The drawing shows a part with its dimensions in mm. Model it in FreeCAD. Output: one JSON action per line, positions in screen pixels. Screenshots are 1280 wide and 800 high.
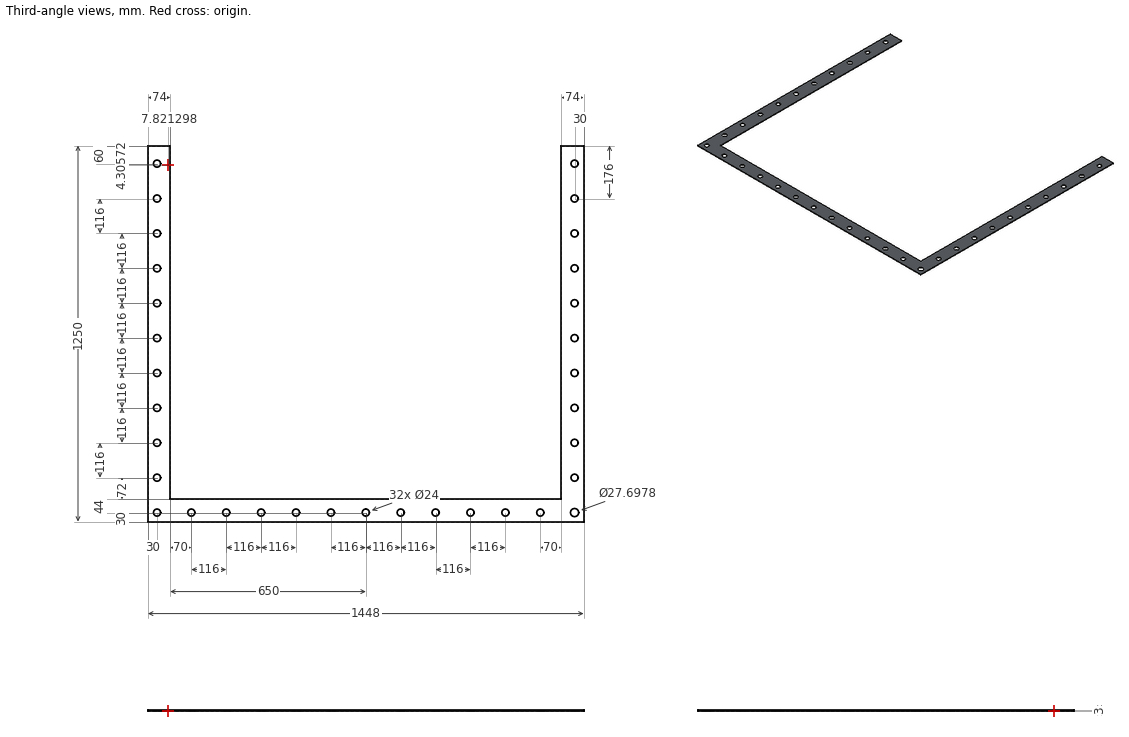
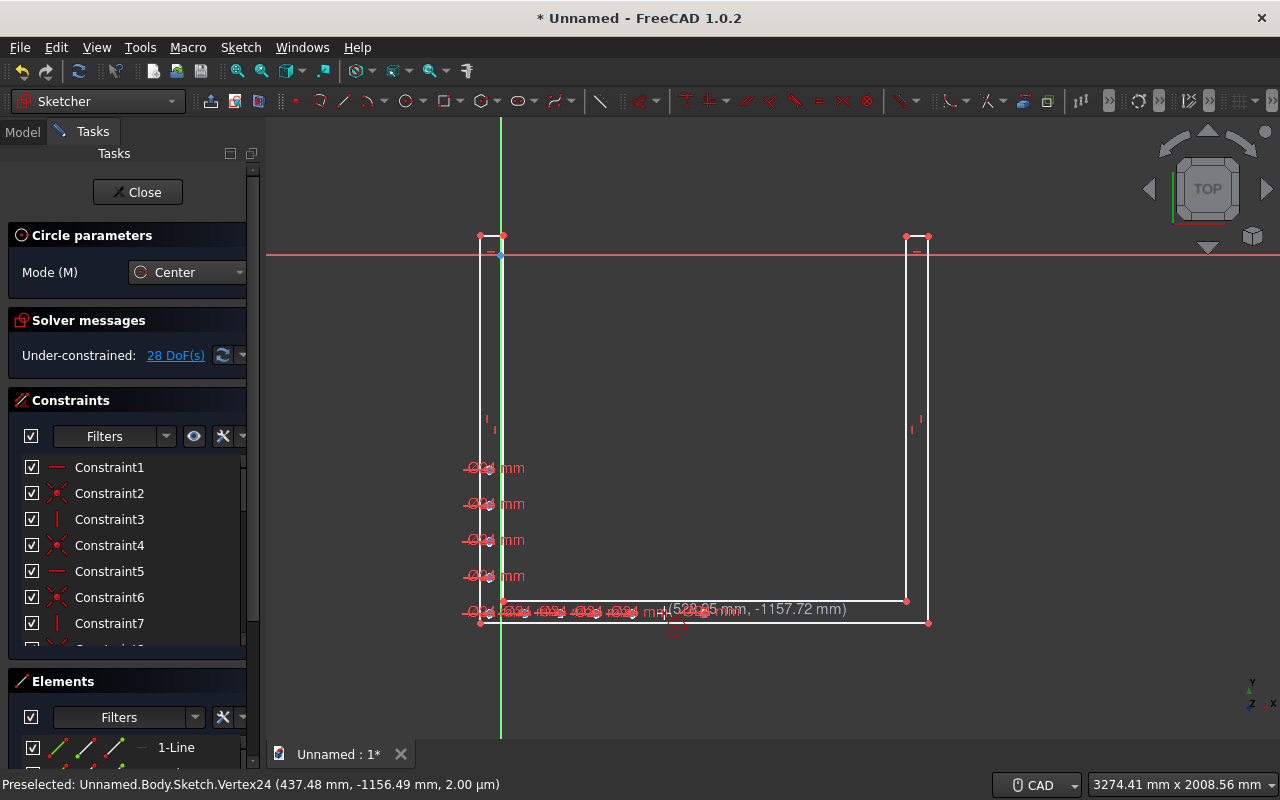
{"action": "scroll", "coordinate": [669, 613], "scroll_direction": "up", "scroll_amount": 3}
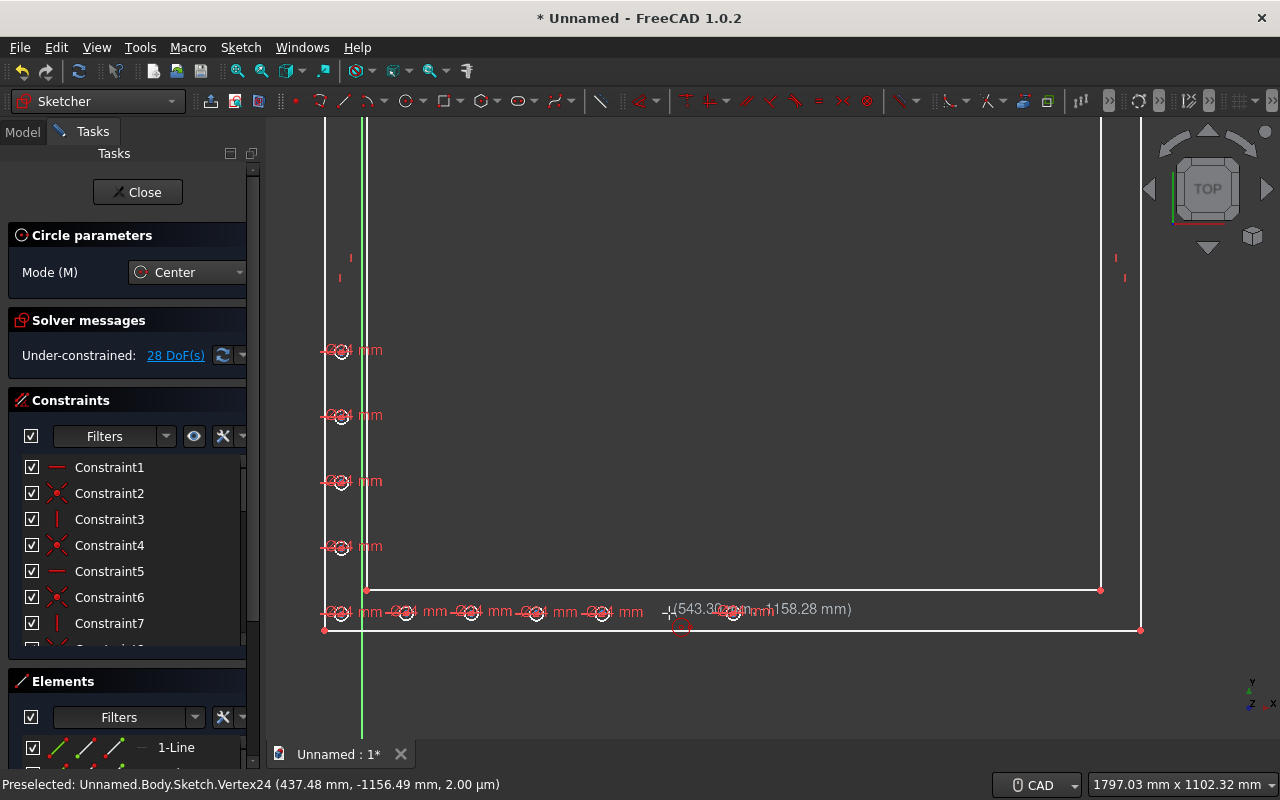
{"action": "left_click", "coordinate": [668, 613]}
{"action": "mouse_move", "coordinate": [673, 608]}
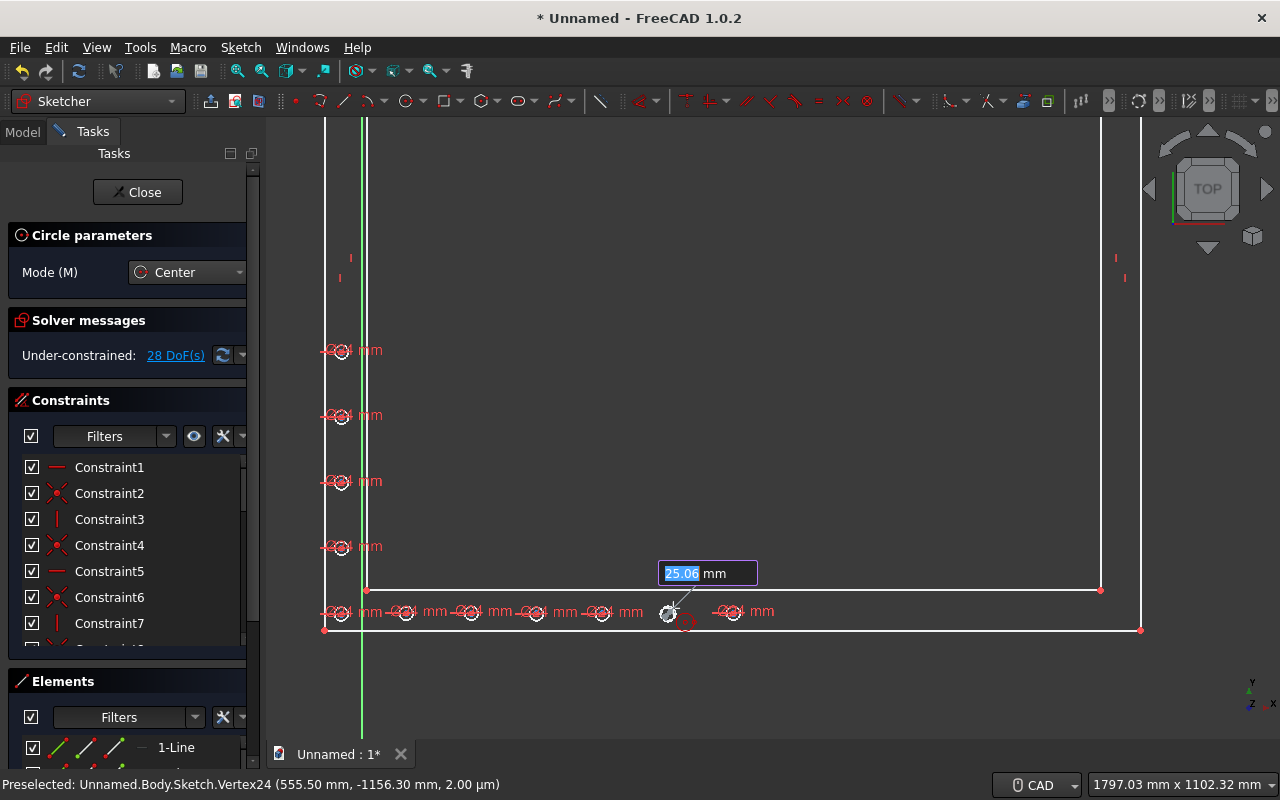
{"action": "type", "text": "24"}
{"action": "key", "text": "Return"}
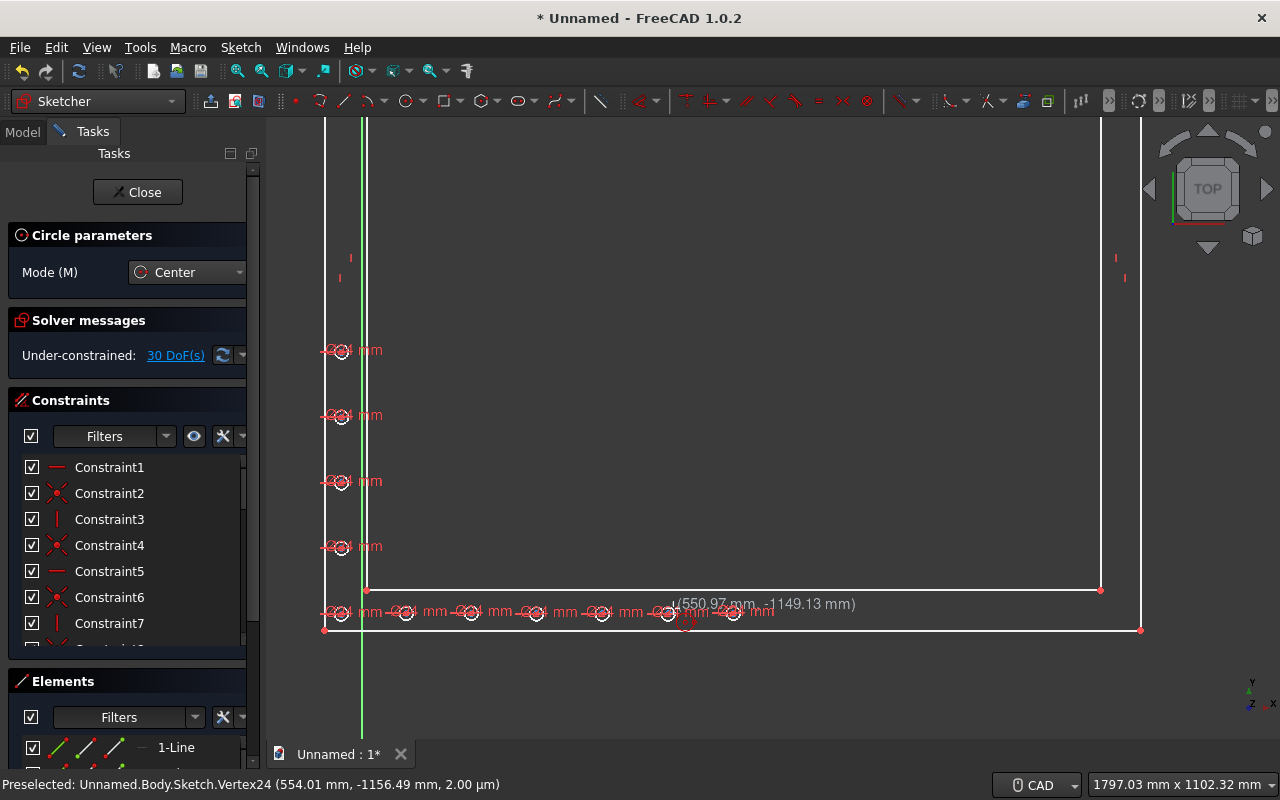
{"action": "scroll", "coordinate": [342, 285], "scroll_direction": "up", "scroll_amount": 7}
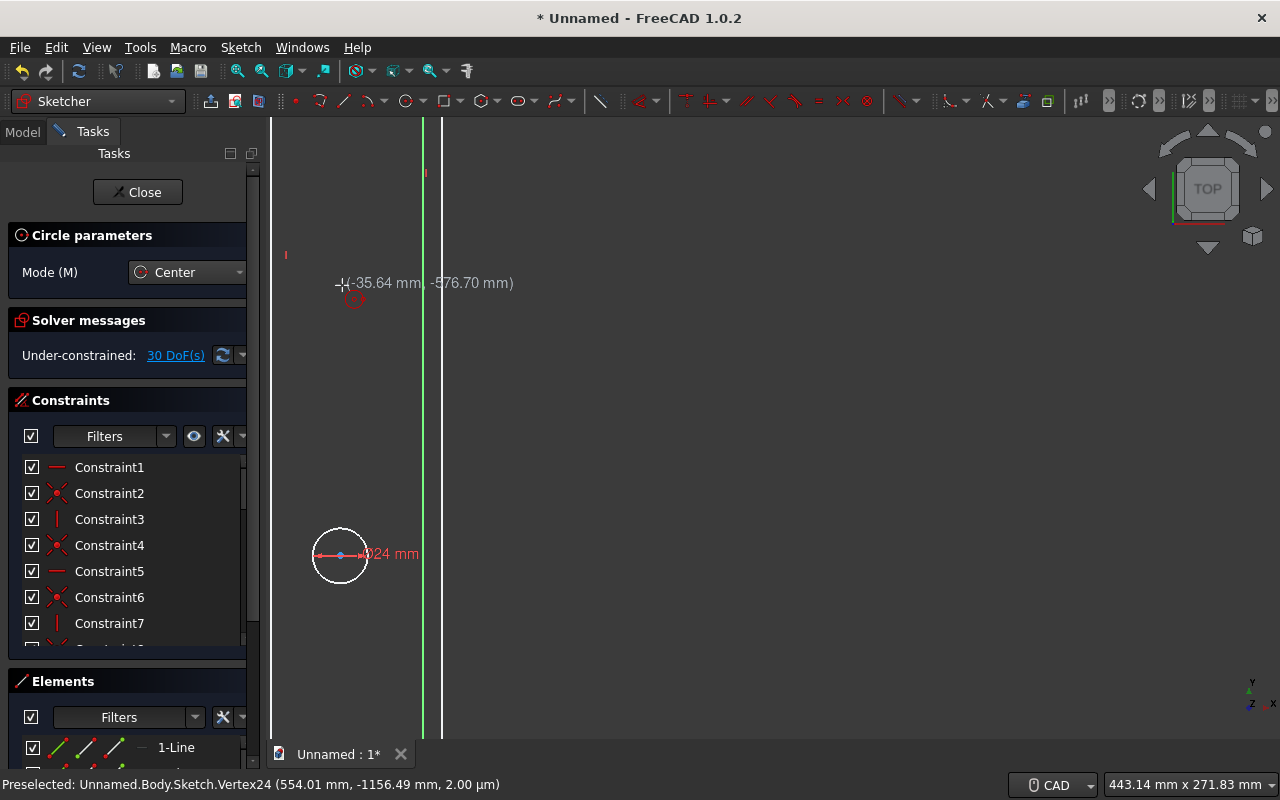
{"action": "scroll", "coordinate": [513, 456], "scroll_direction": "down", "scroll_amount": 10}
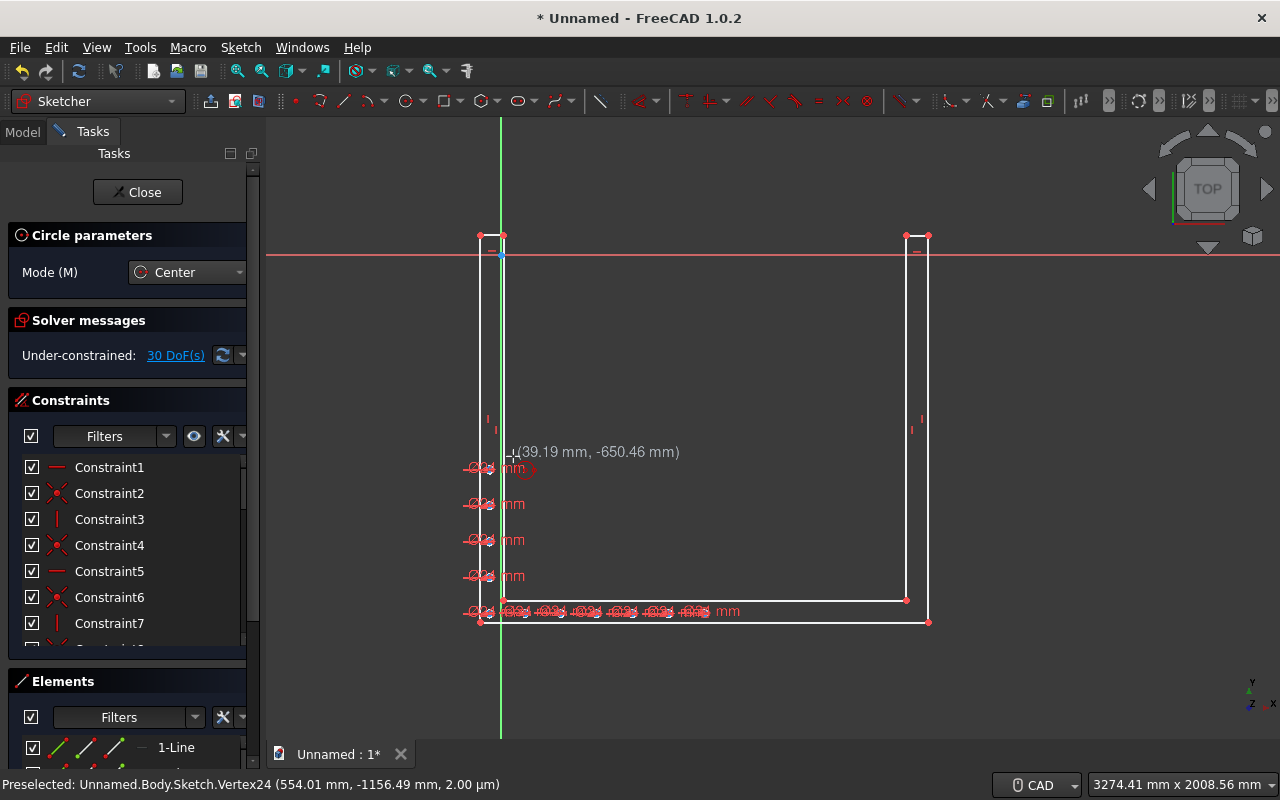
{"action": "scroll", "coordinate": [490, 433], "scroll_direction": "up", "scroll_amount": 3}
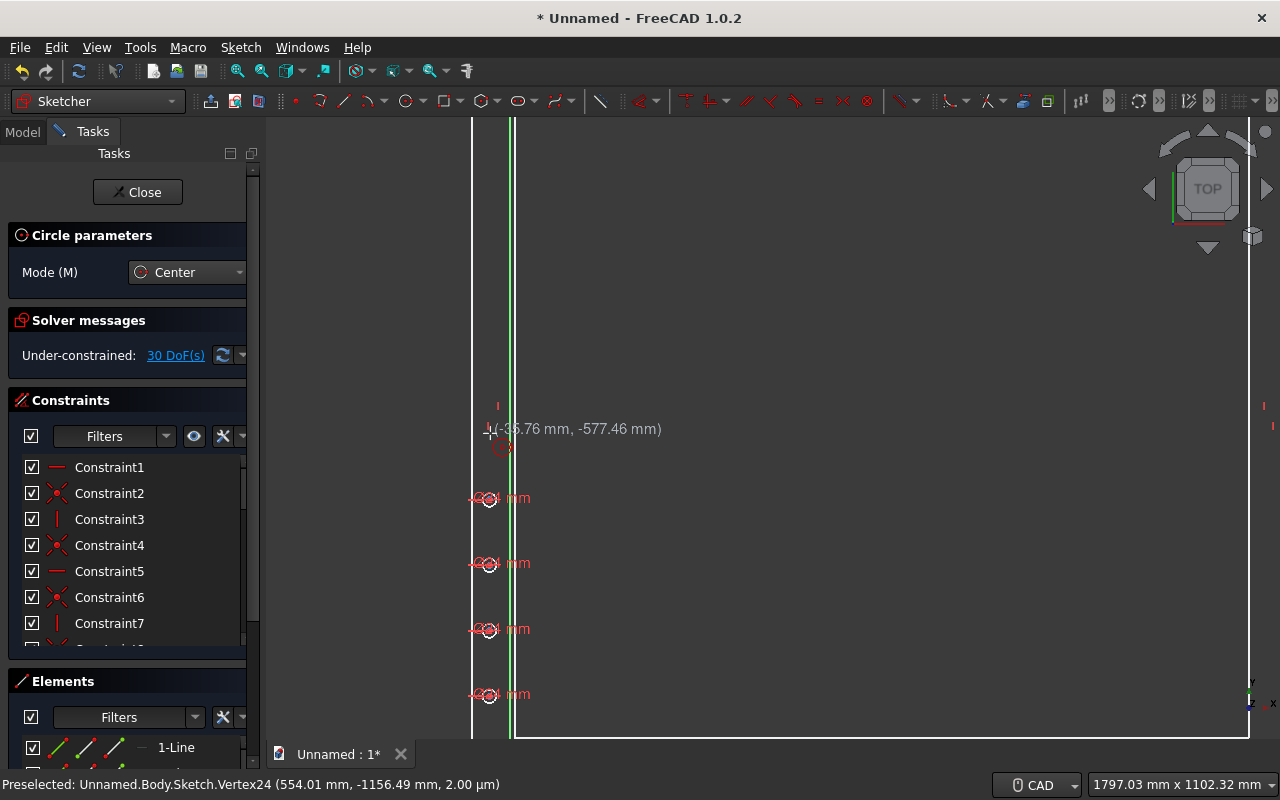
{"action": "left_click", "coordinate": [490, 433]}
{"action": "mouse_move", "coordinate": [494, 429]}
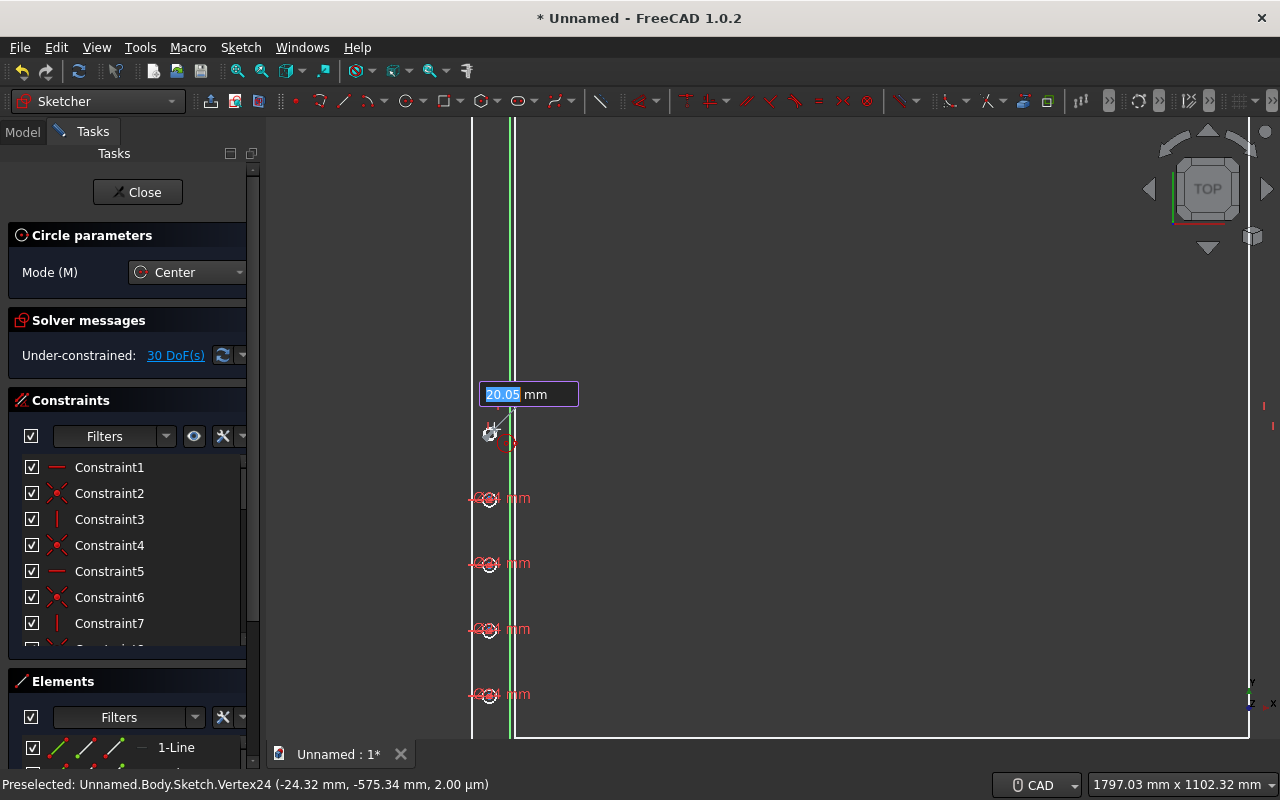
{"action": "type", "text": "24"}
{"action": "key", "text": "Return"}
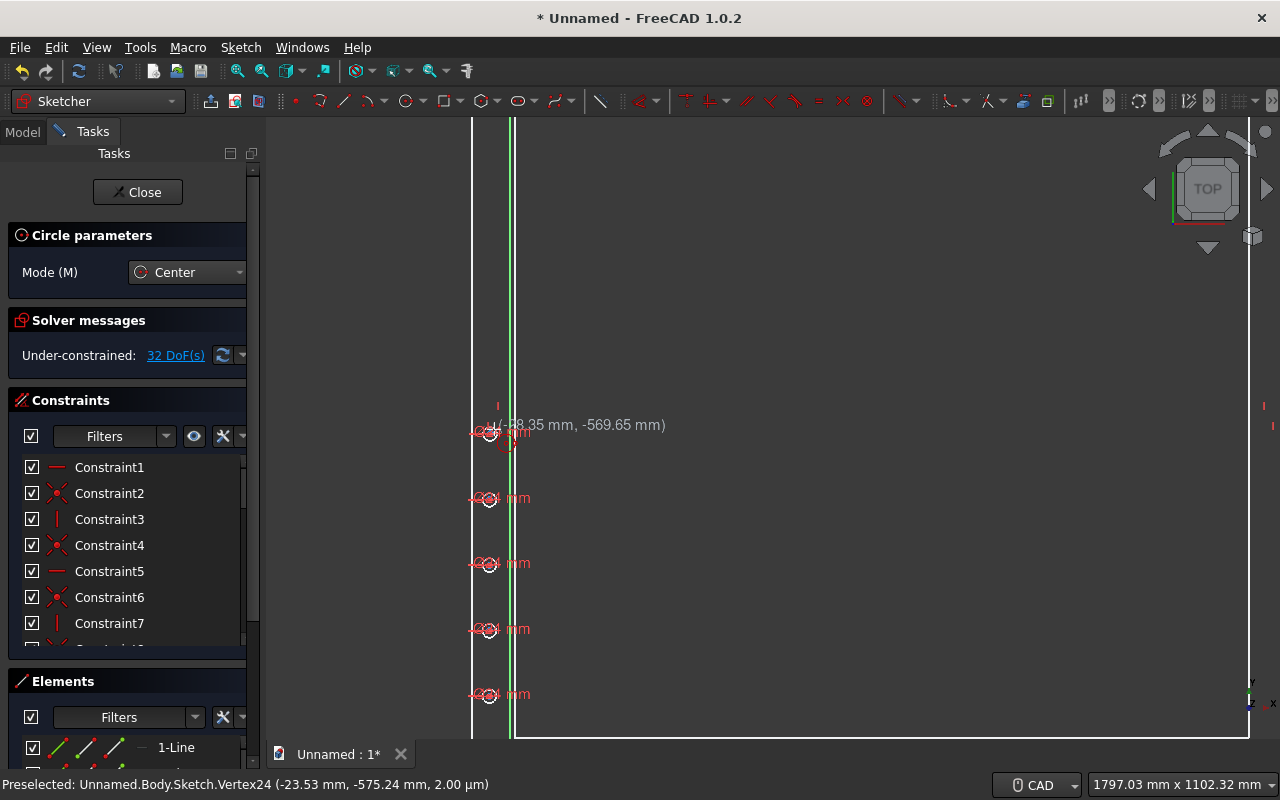
{"action": "scroll", "coordinate": [490, 368], "scroll_direction": "up", "scroll_amount": 7}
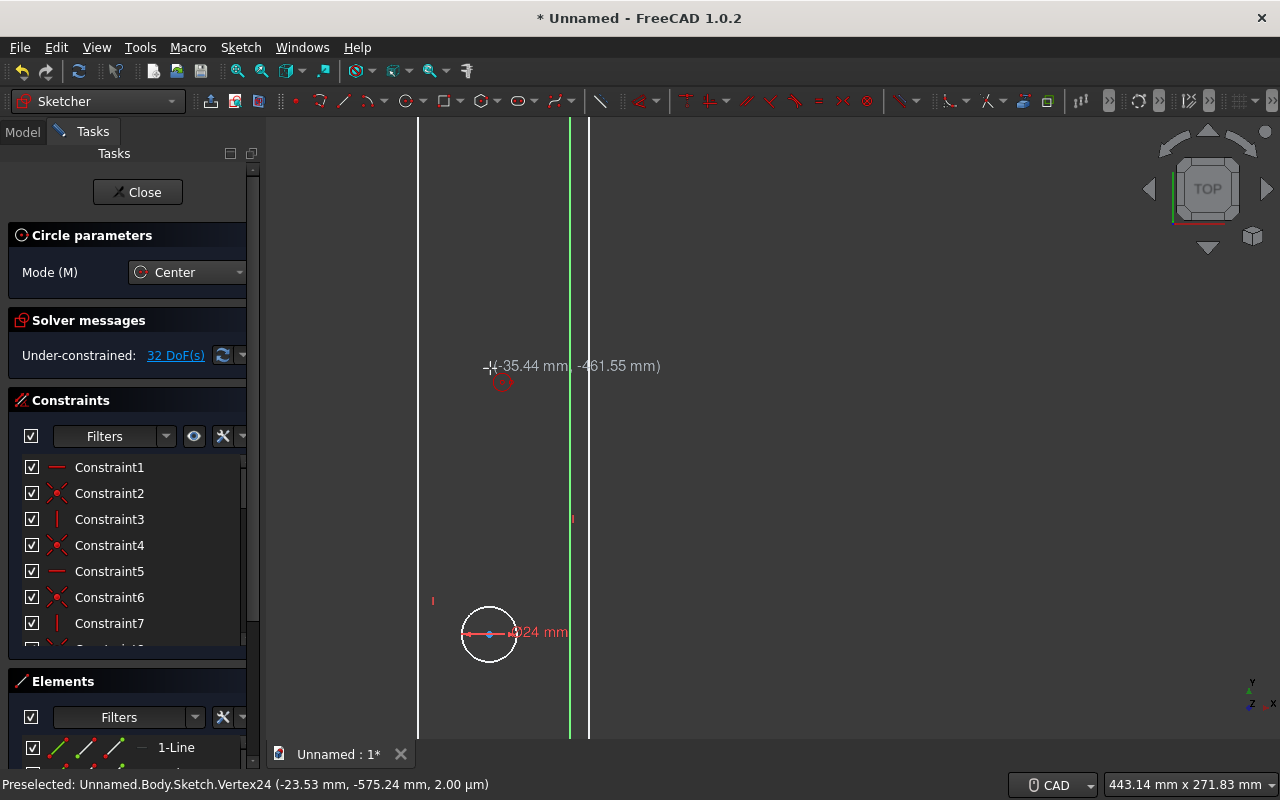
{"action": "scroll", "coordinate": [490, 401], "scroll_direction": "down", "scroll_amount": 10}